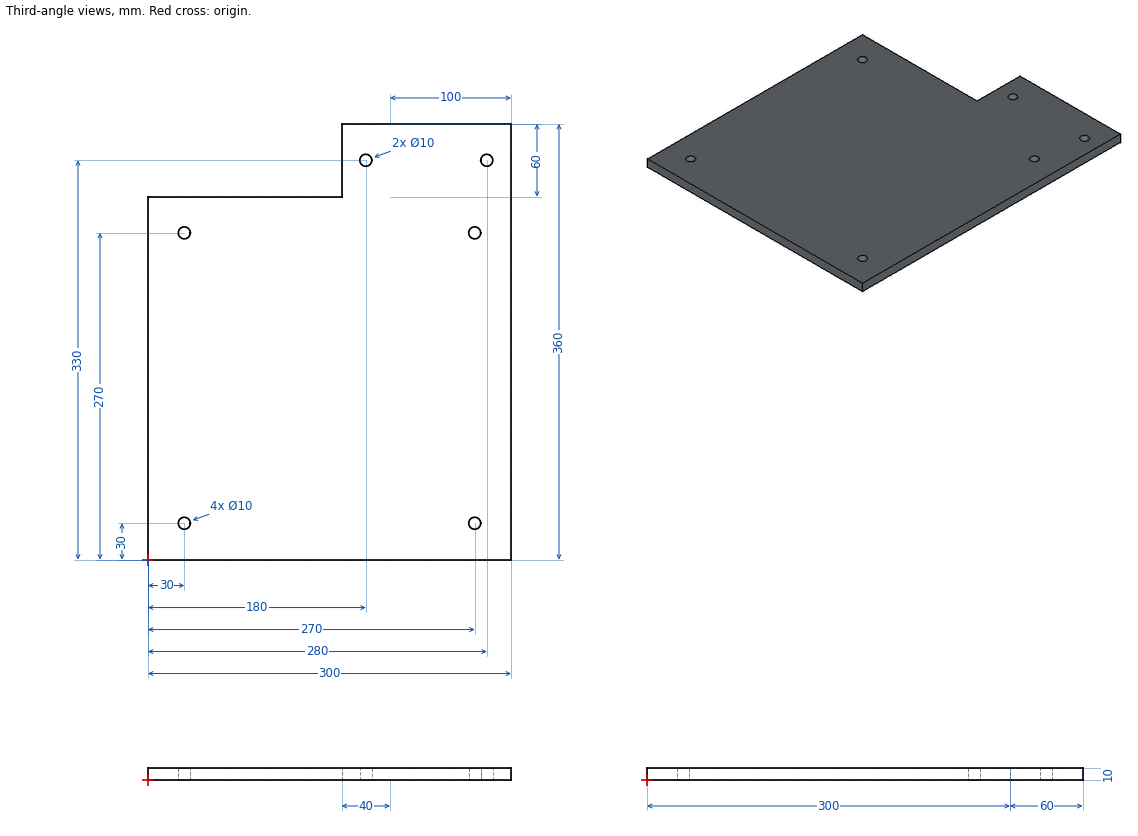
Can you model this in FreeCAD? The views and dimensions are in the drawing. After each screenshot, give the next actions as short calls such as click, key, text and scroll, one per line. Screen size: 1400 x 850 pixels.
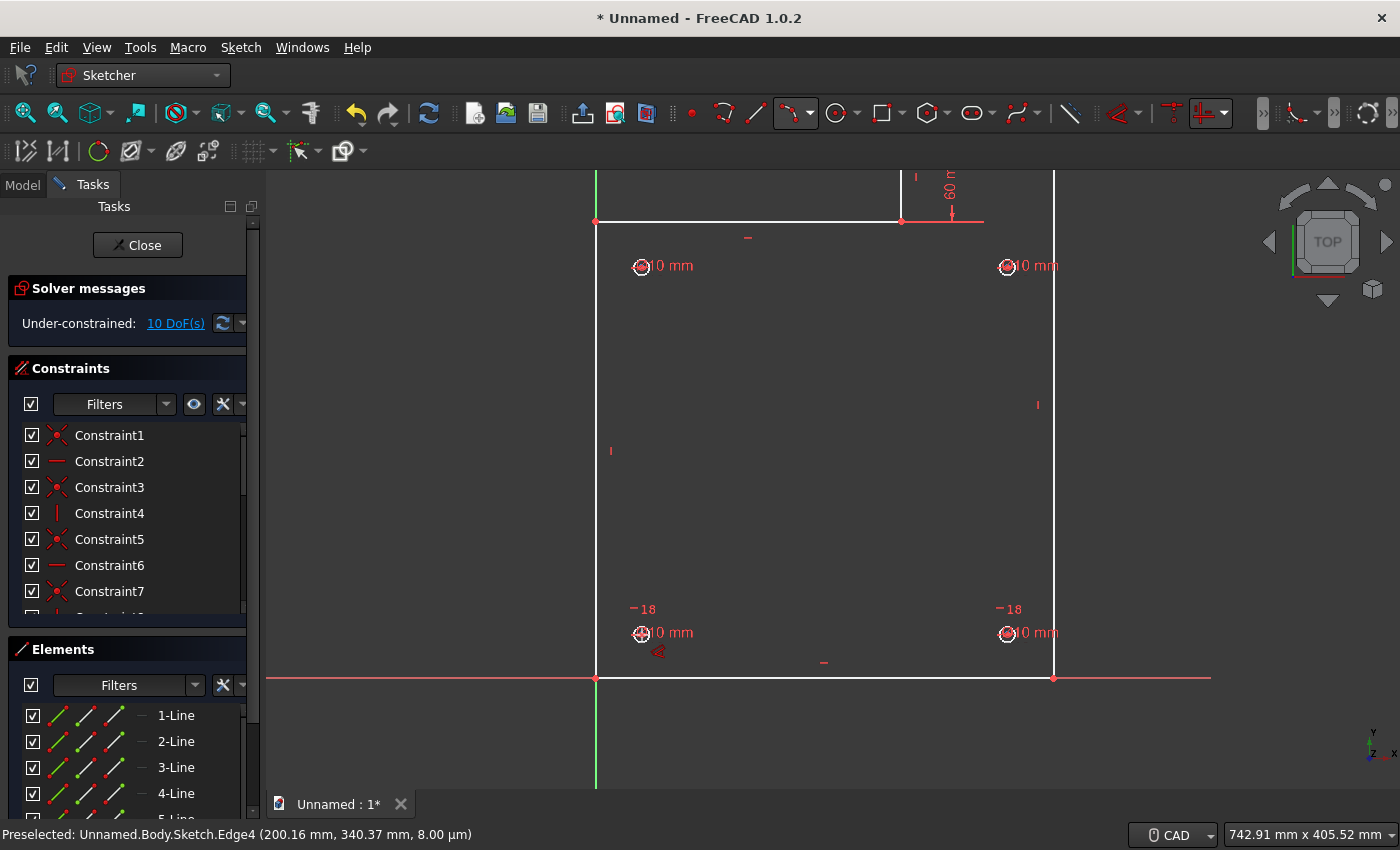
click(642, 635)
click(619, 712)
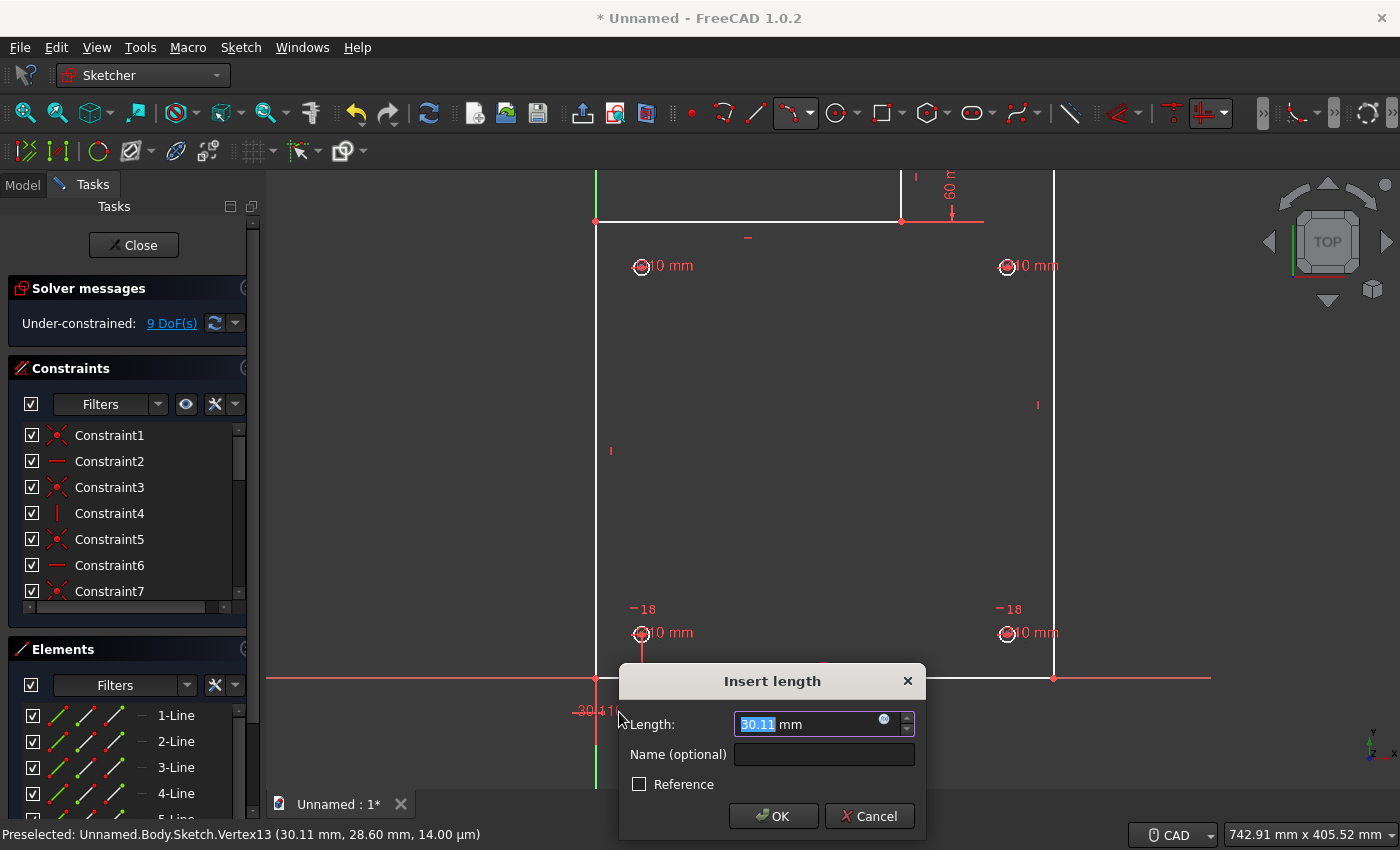
text(30)
key(Return)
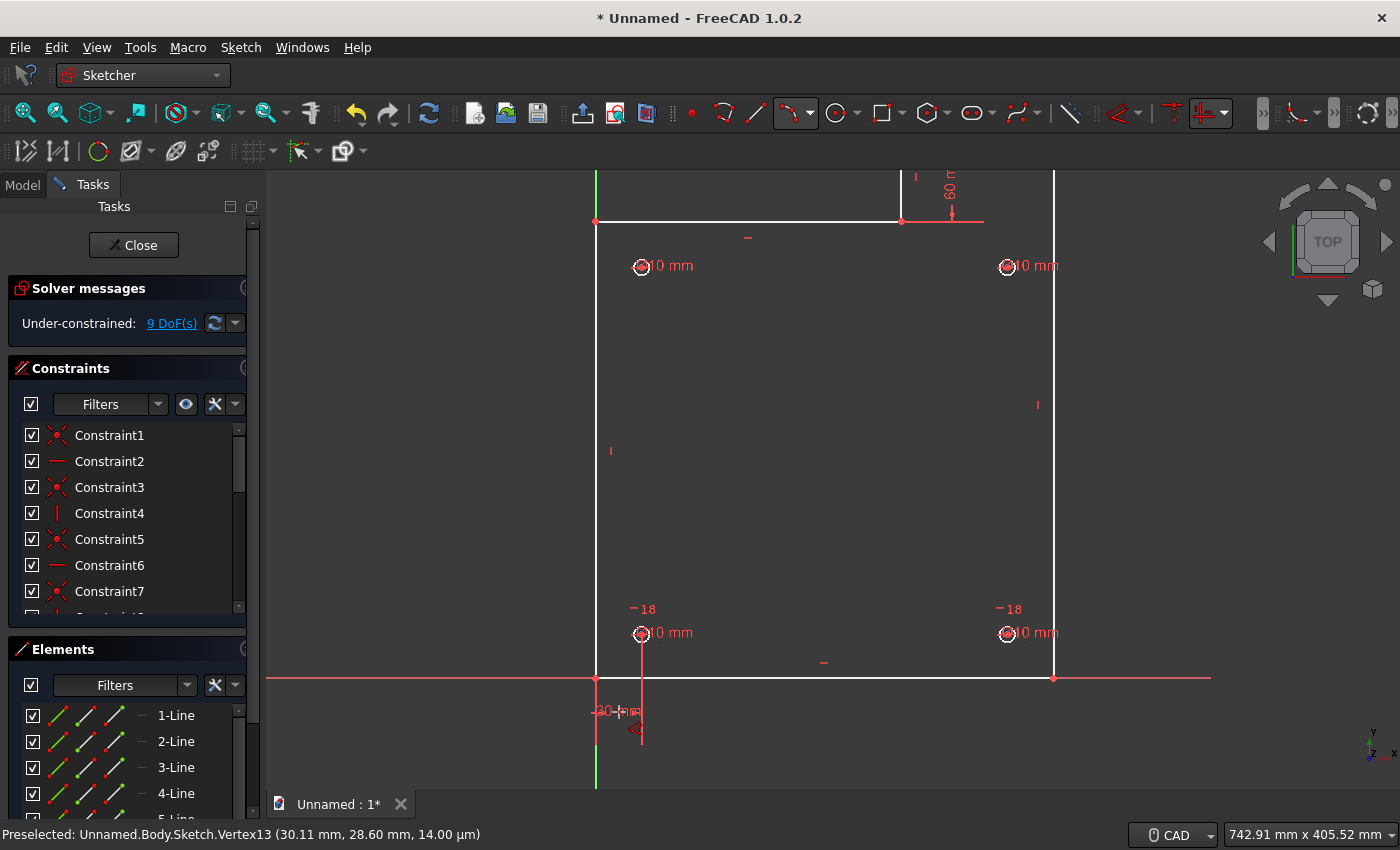
click(642, 635)
click(562, 656)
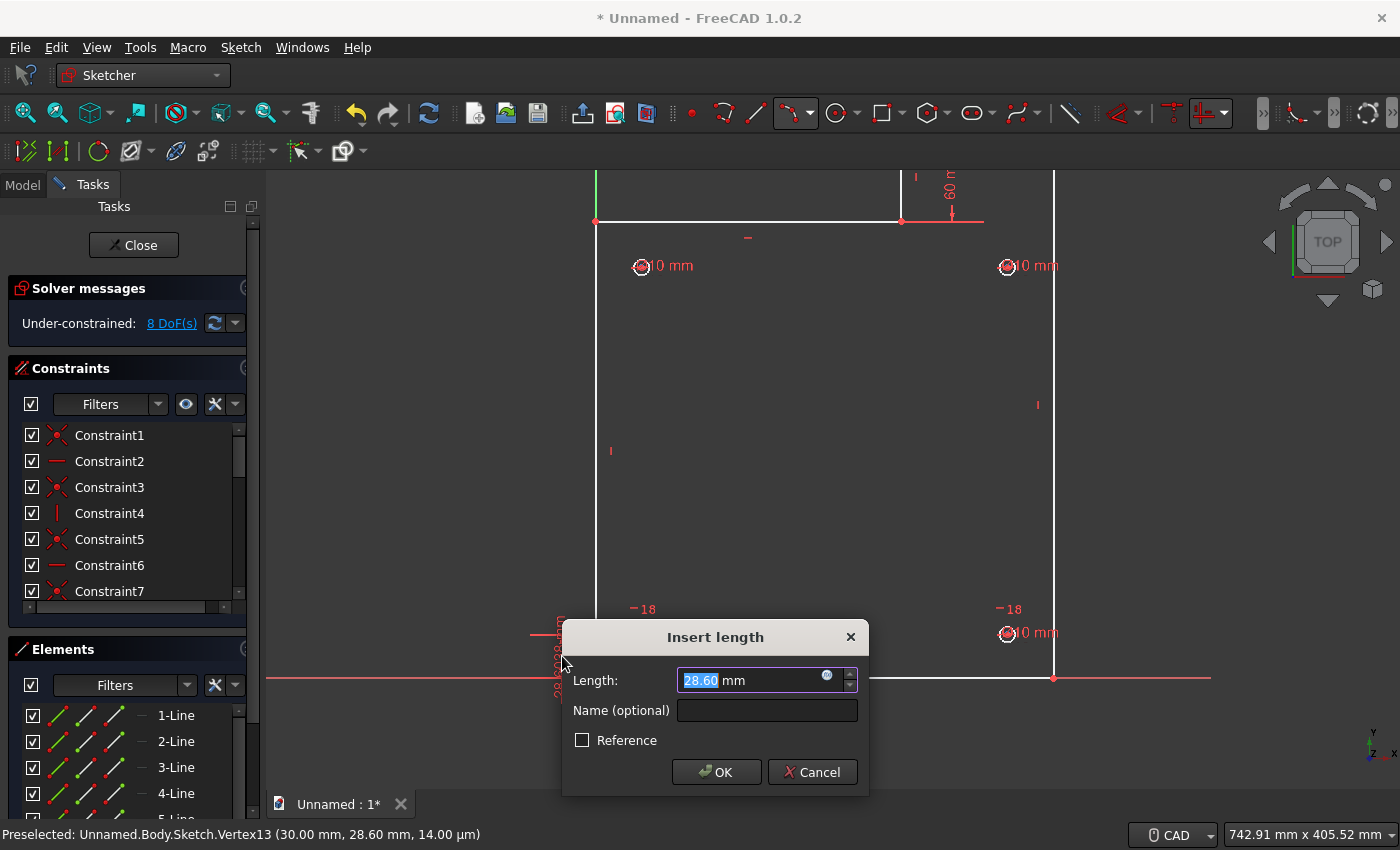
text(30)
key(Return)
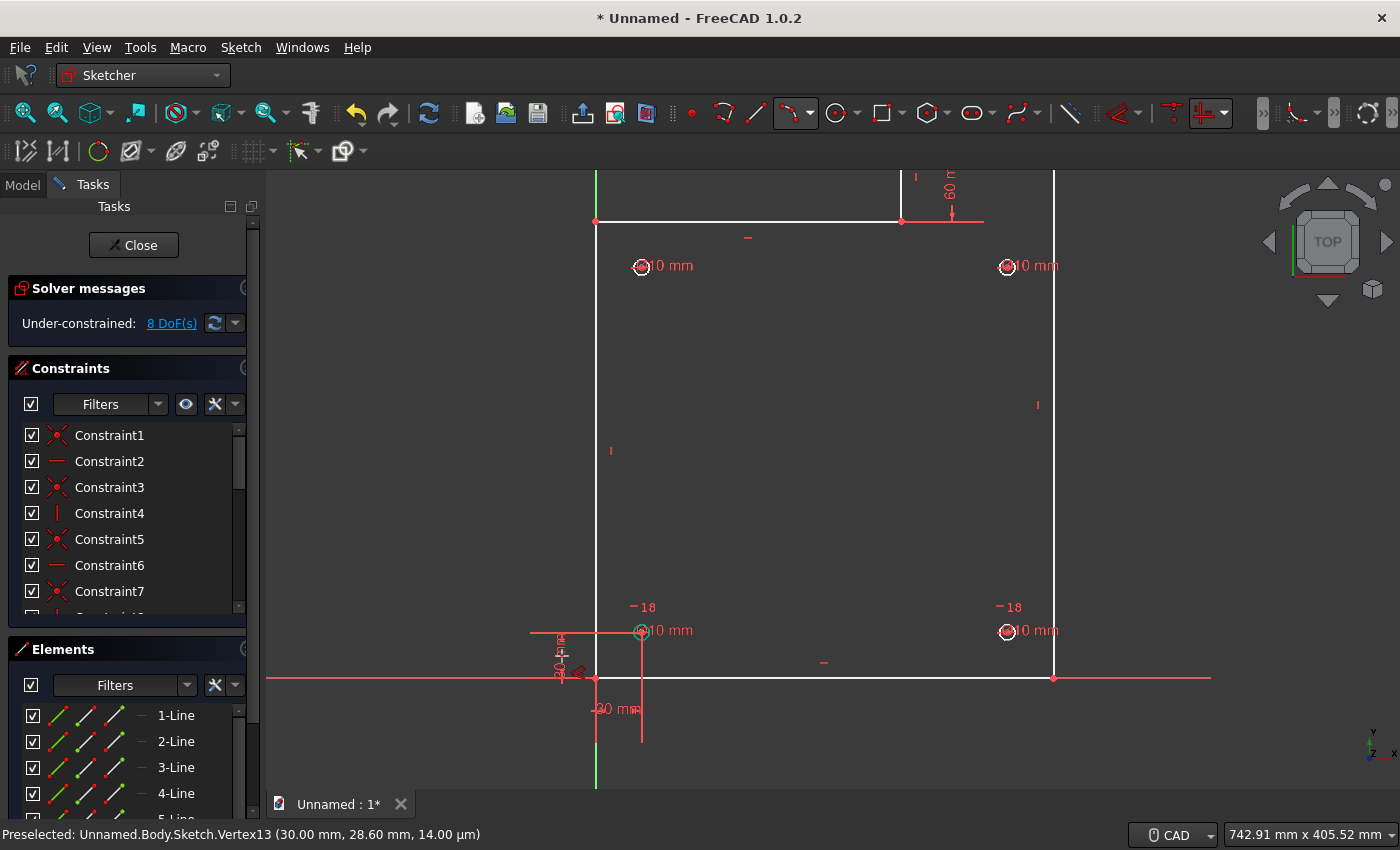
click(642, 268)
click(619, 736)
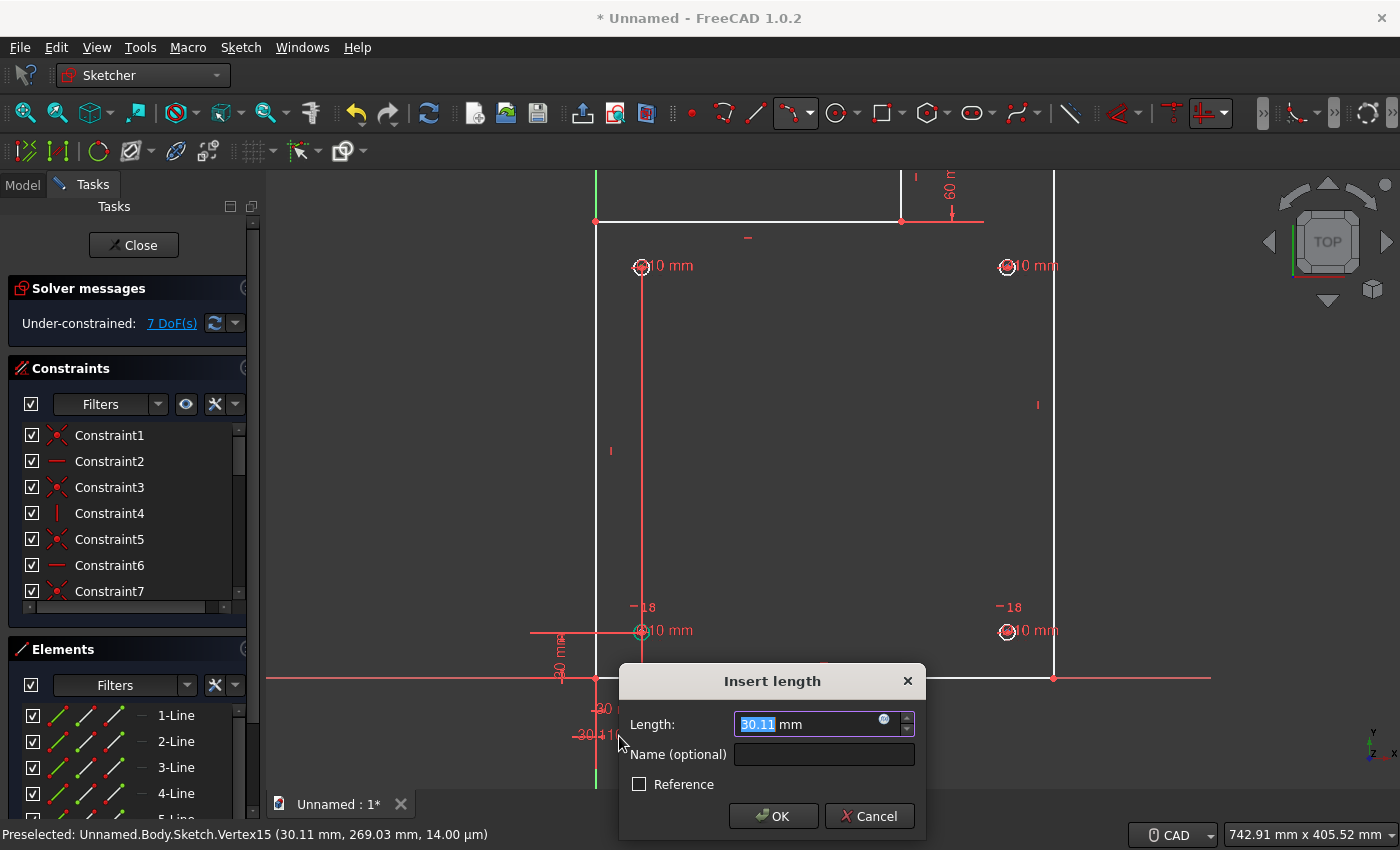
text(30)
key(Return)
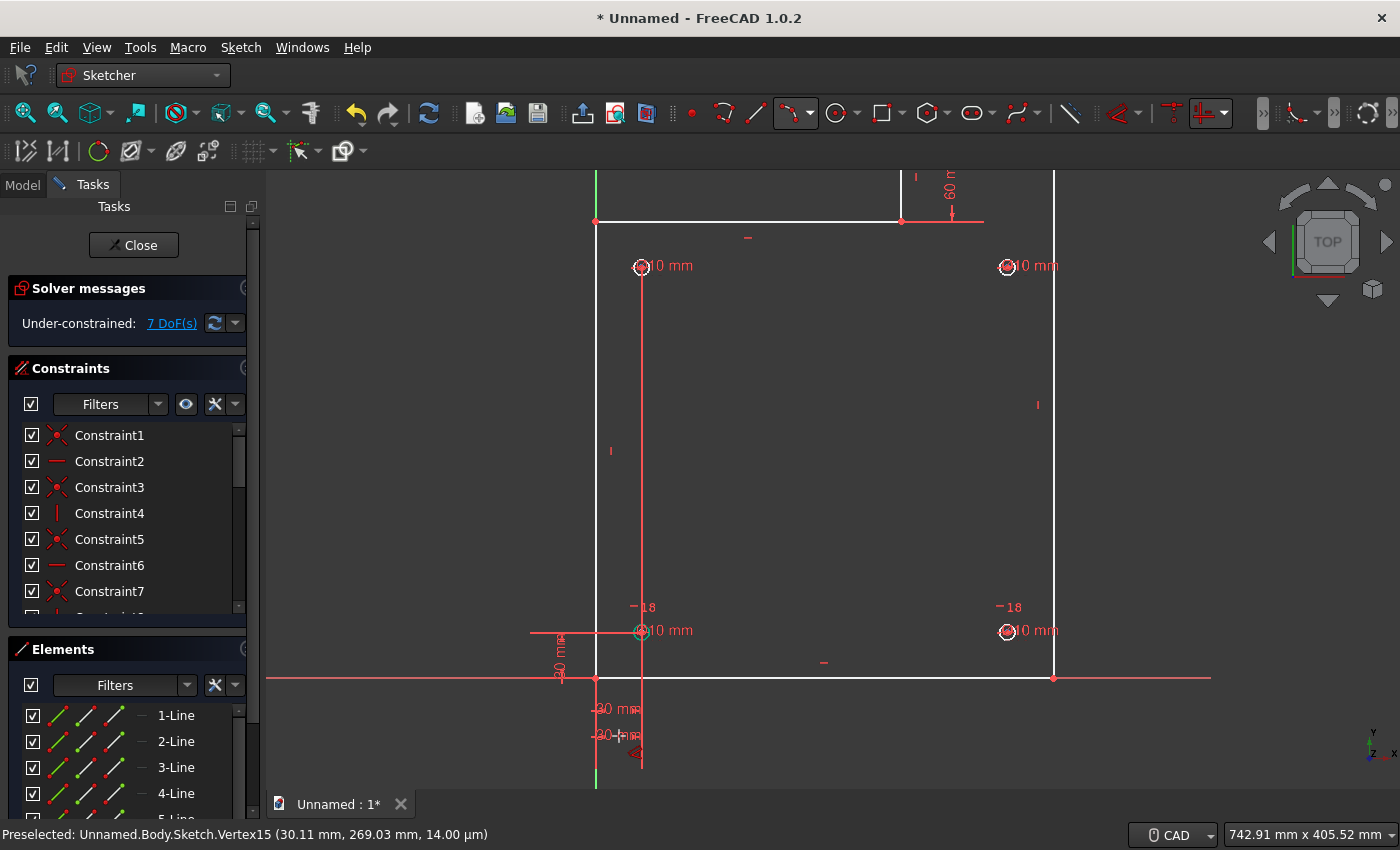
click(733, 678)
click(825, 712)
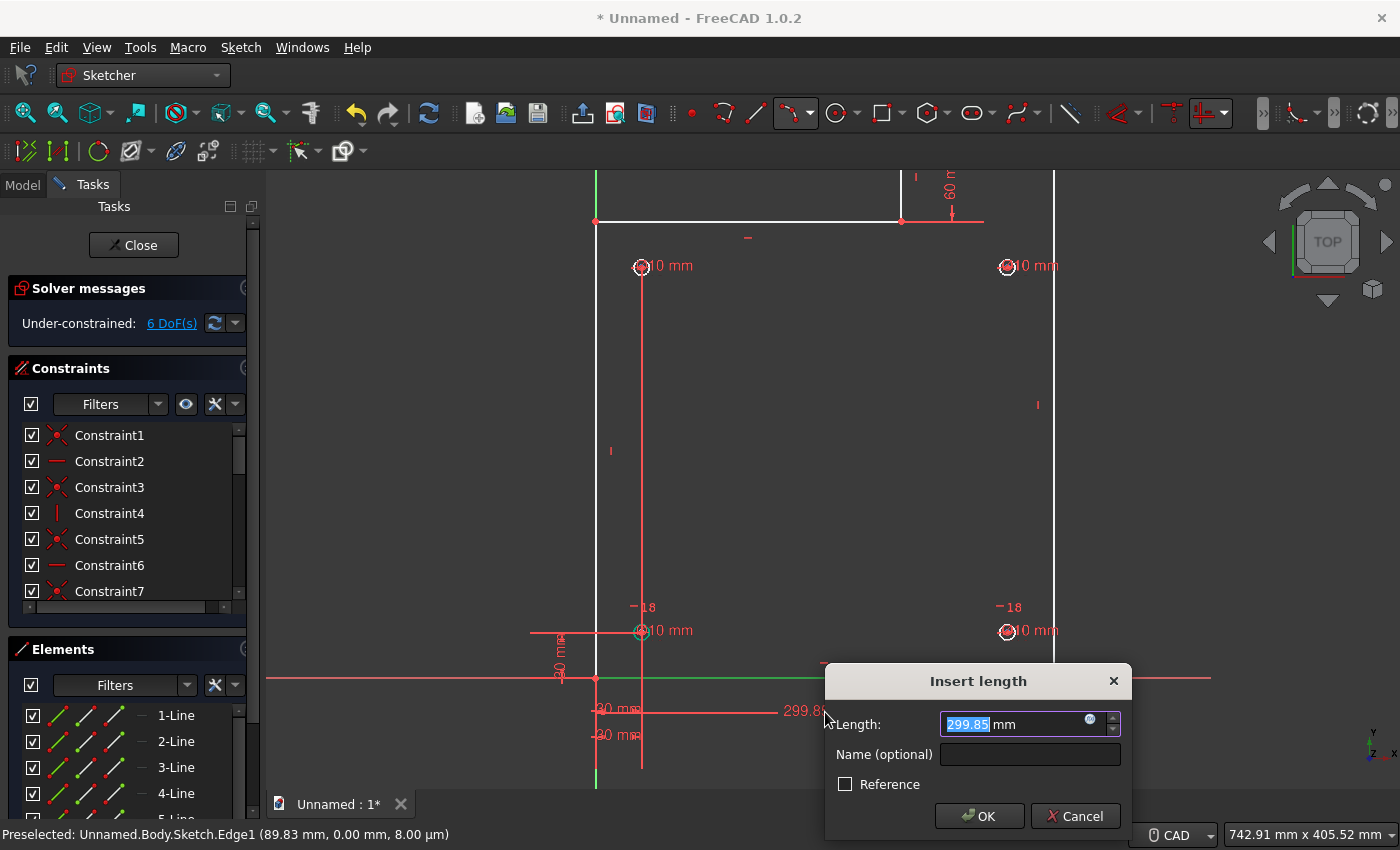
text(300)
key(Return)